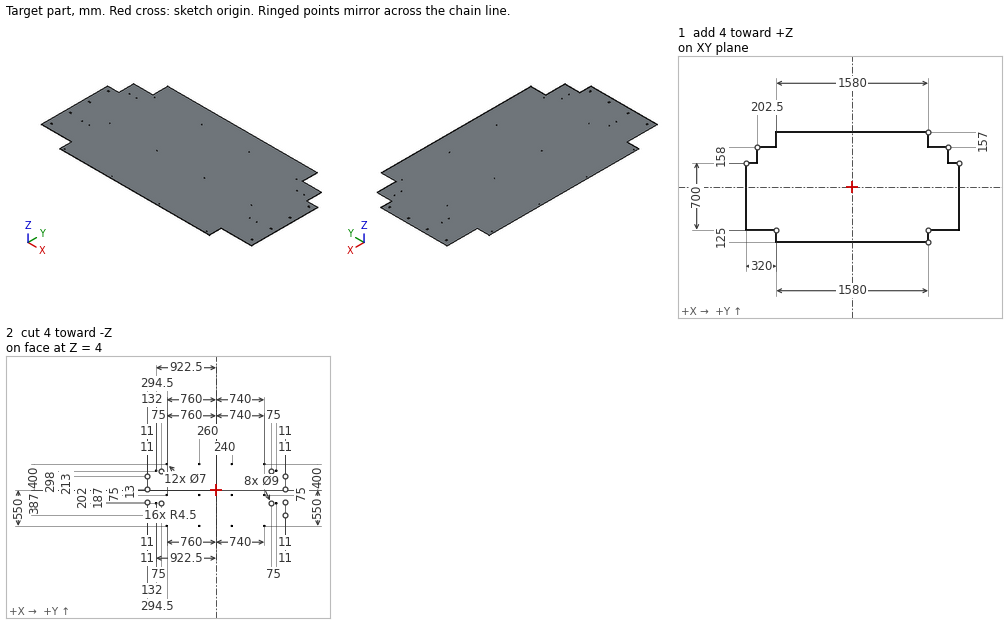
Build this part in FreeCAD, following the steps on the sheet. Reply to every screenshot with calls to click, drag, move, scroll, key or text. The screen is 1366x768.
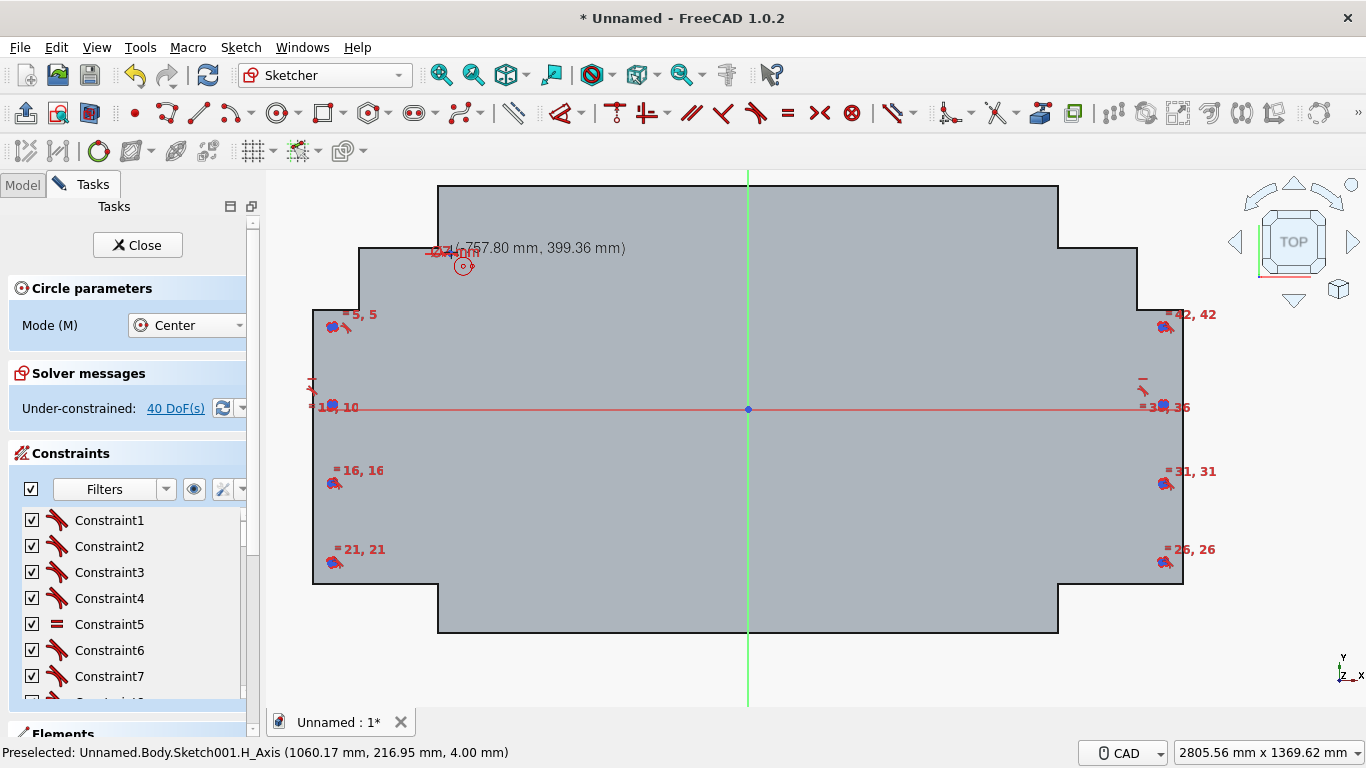
scroll(646, 253, up, 15)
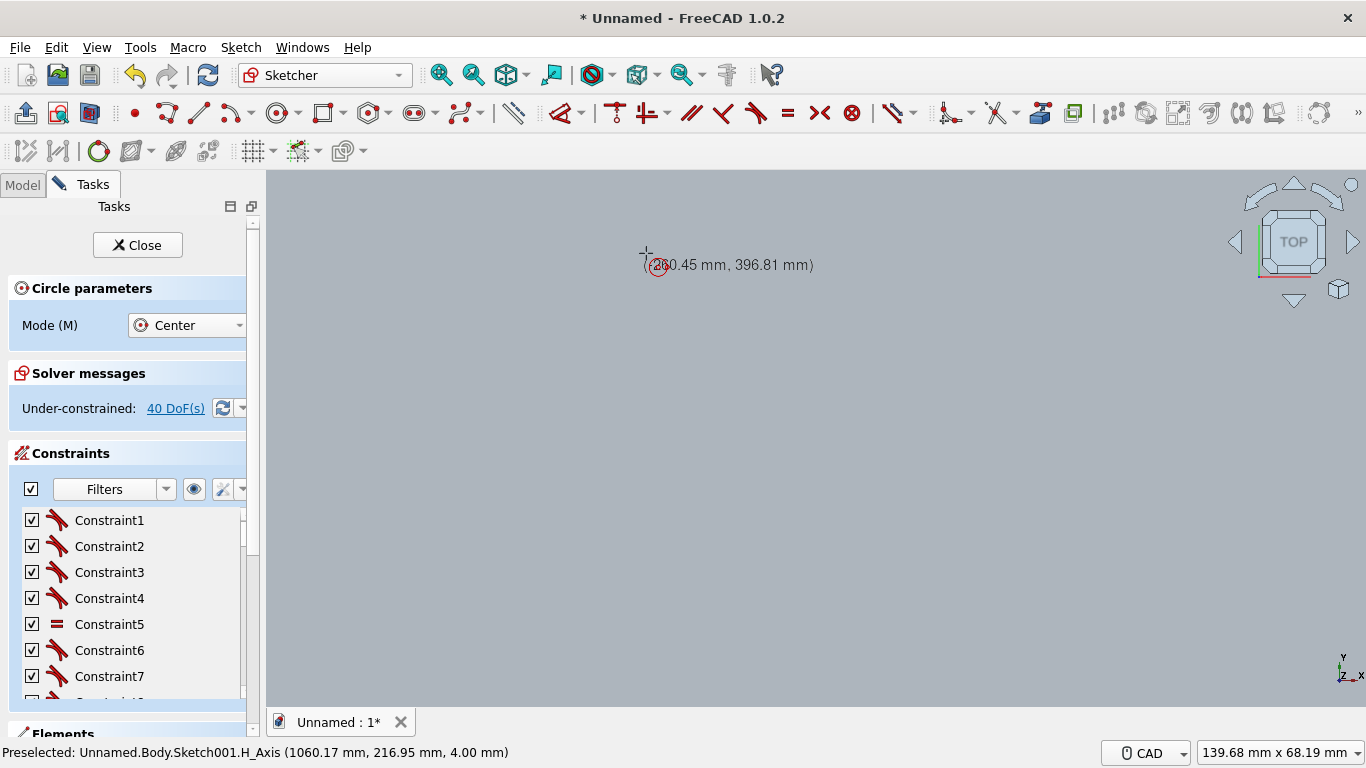
scroll(646, 253, down, 15)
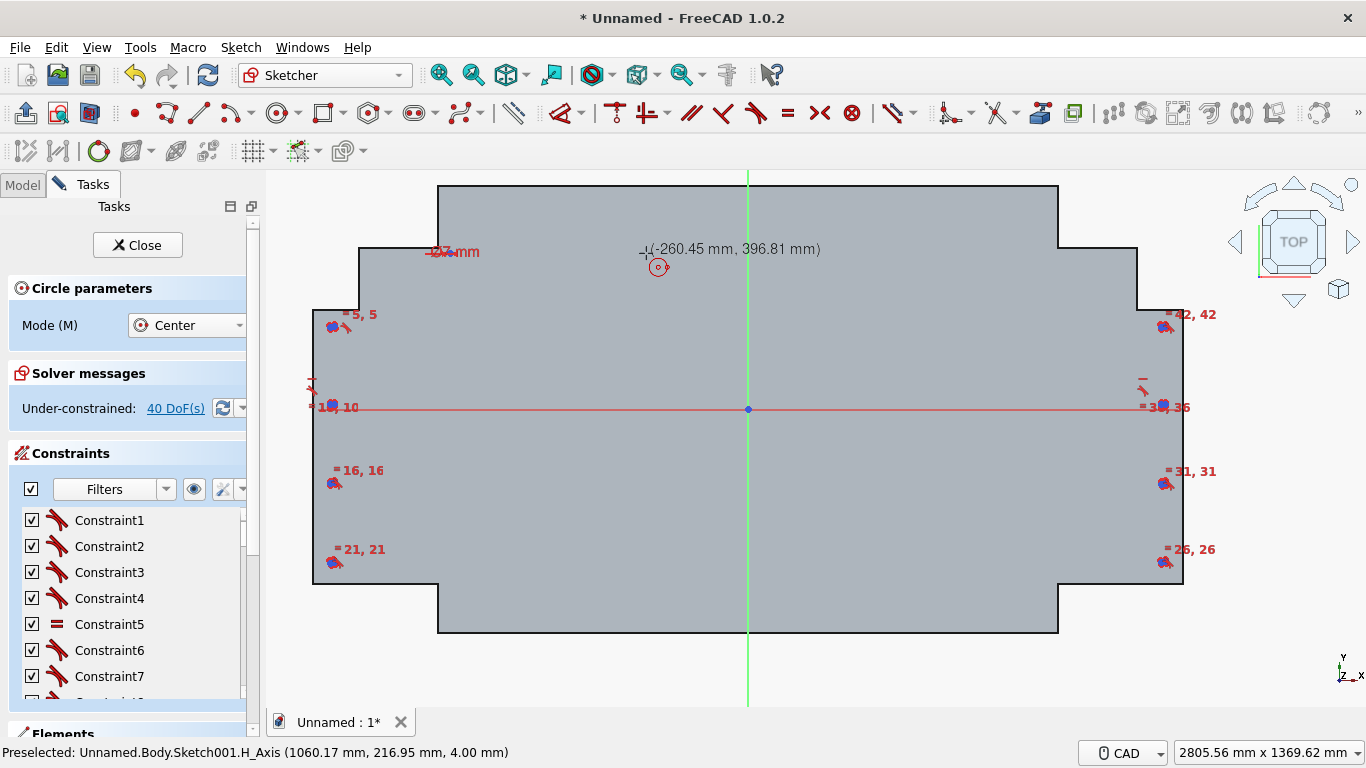
click(646, 253)
move(647, 252)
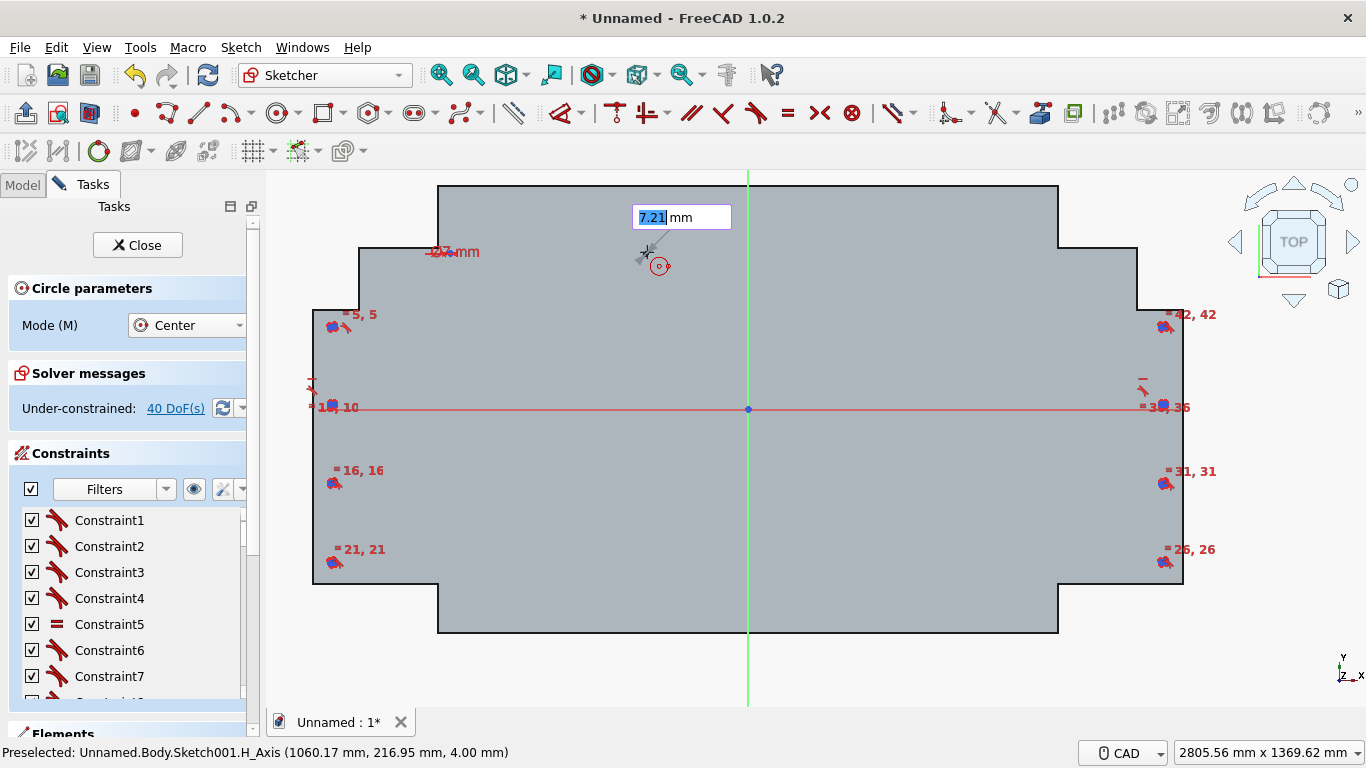
text(7)
key(Return)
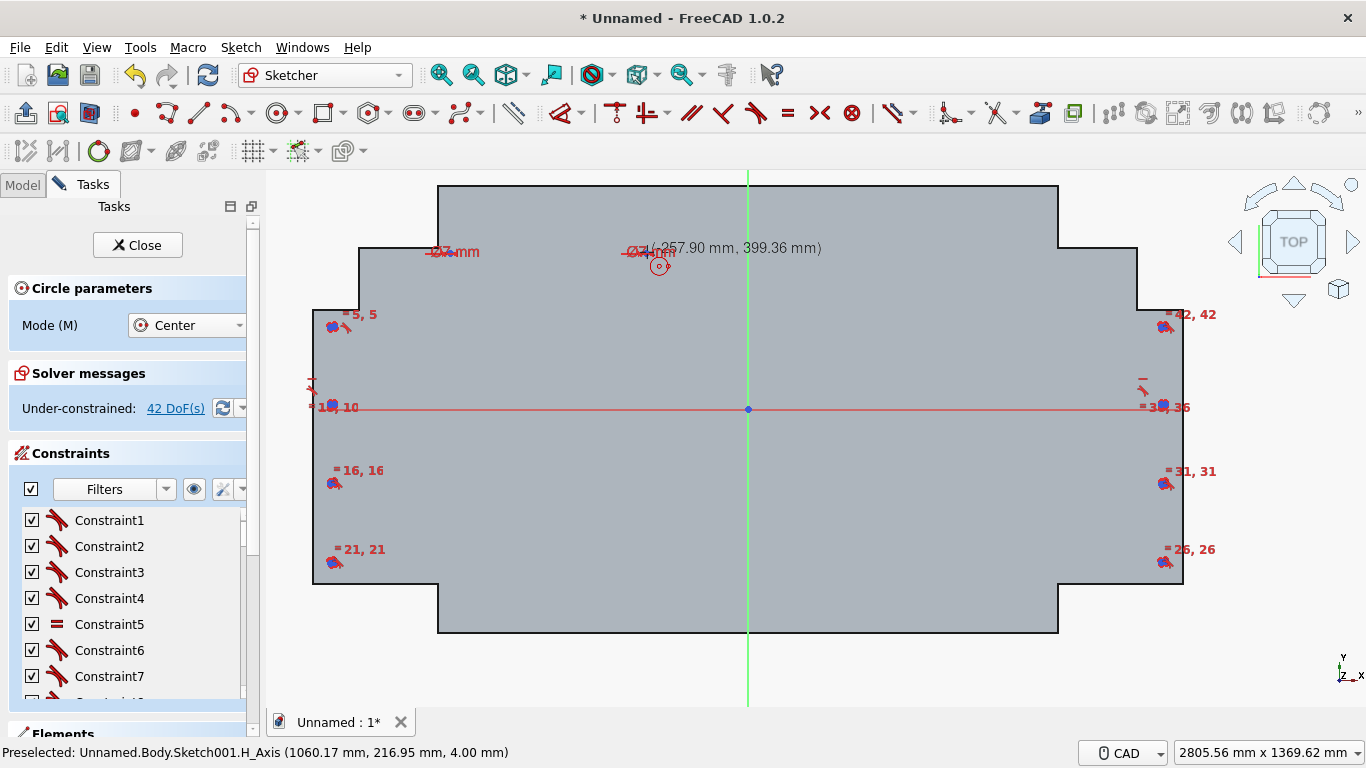
scroll(842, 253, up, 15)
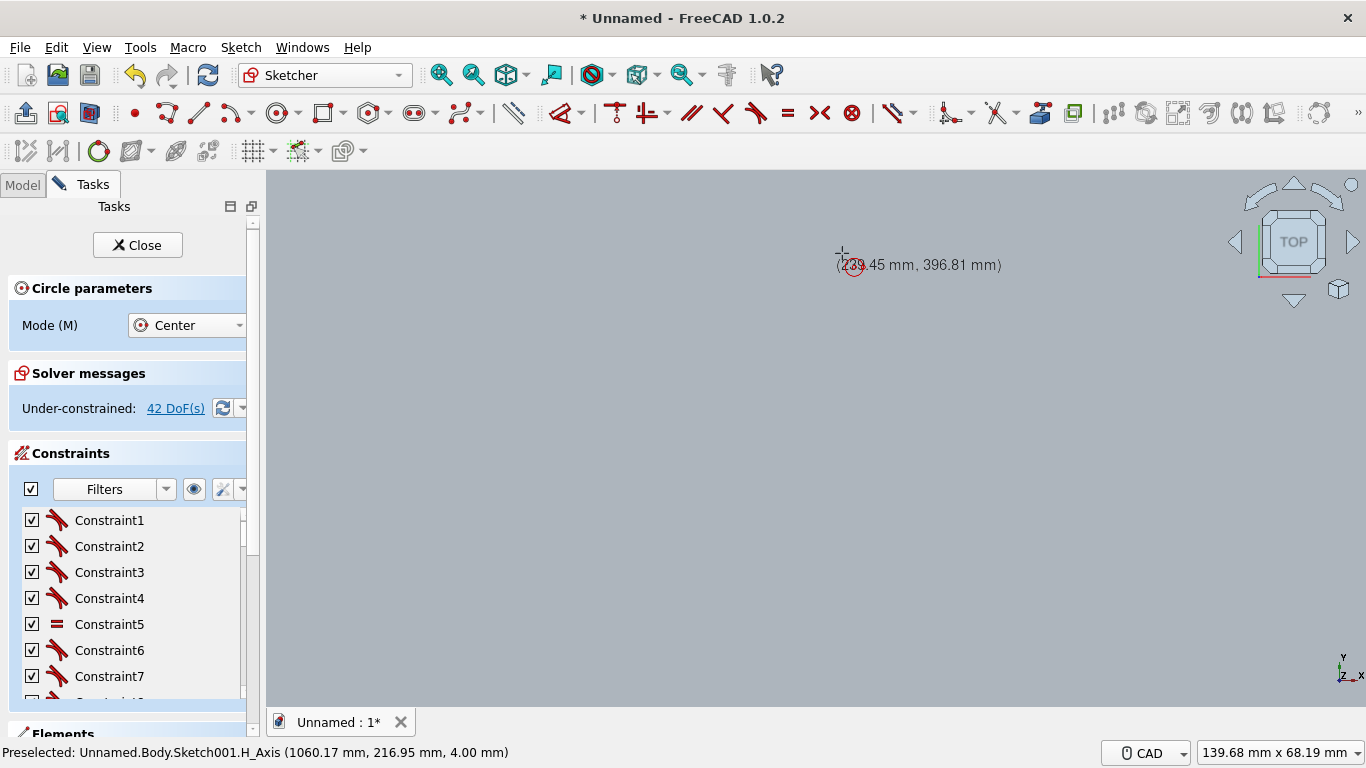
scroll(842, 253, down, 15)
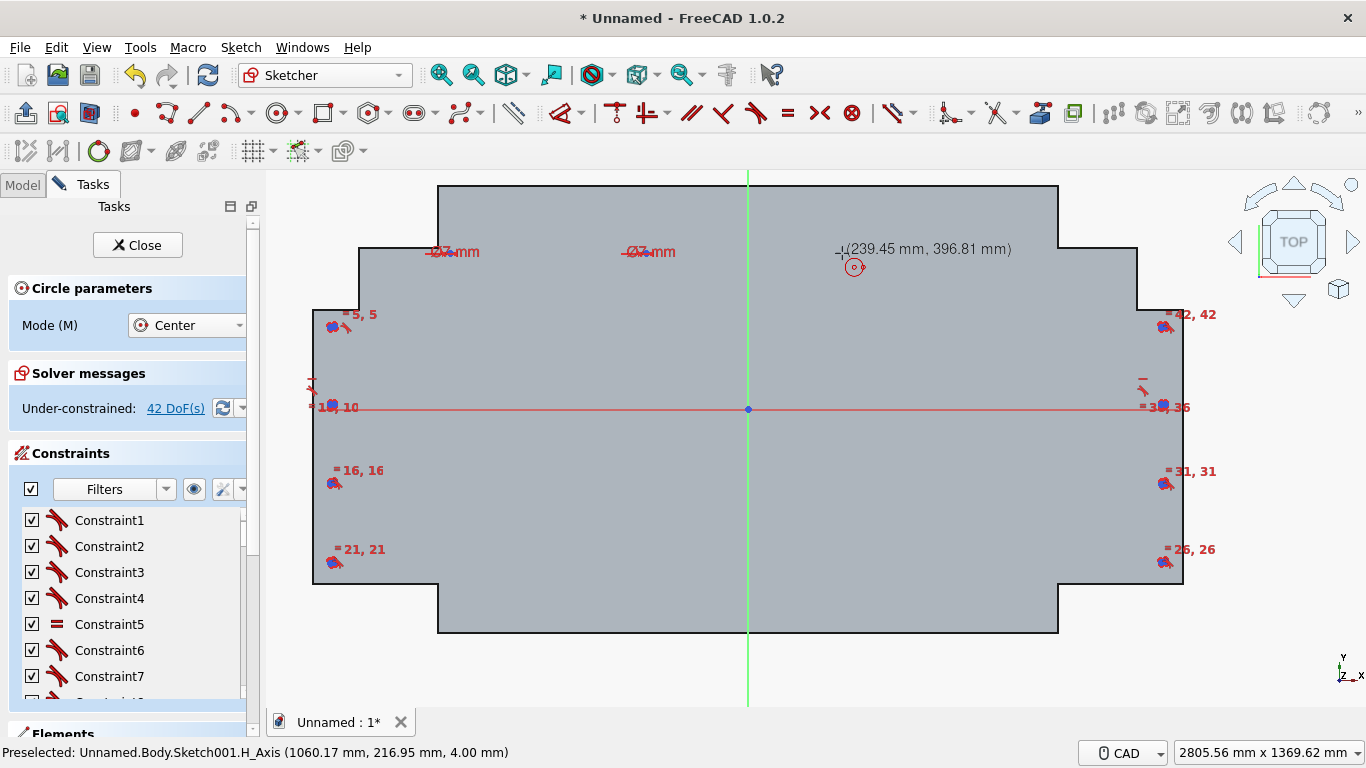
click(842, 253)
move(843, 252)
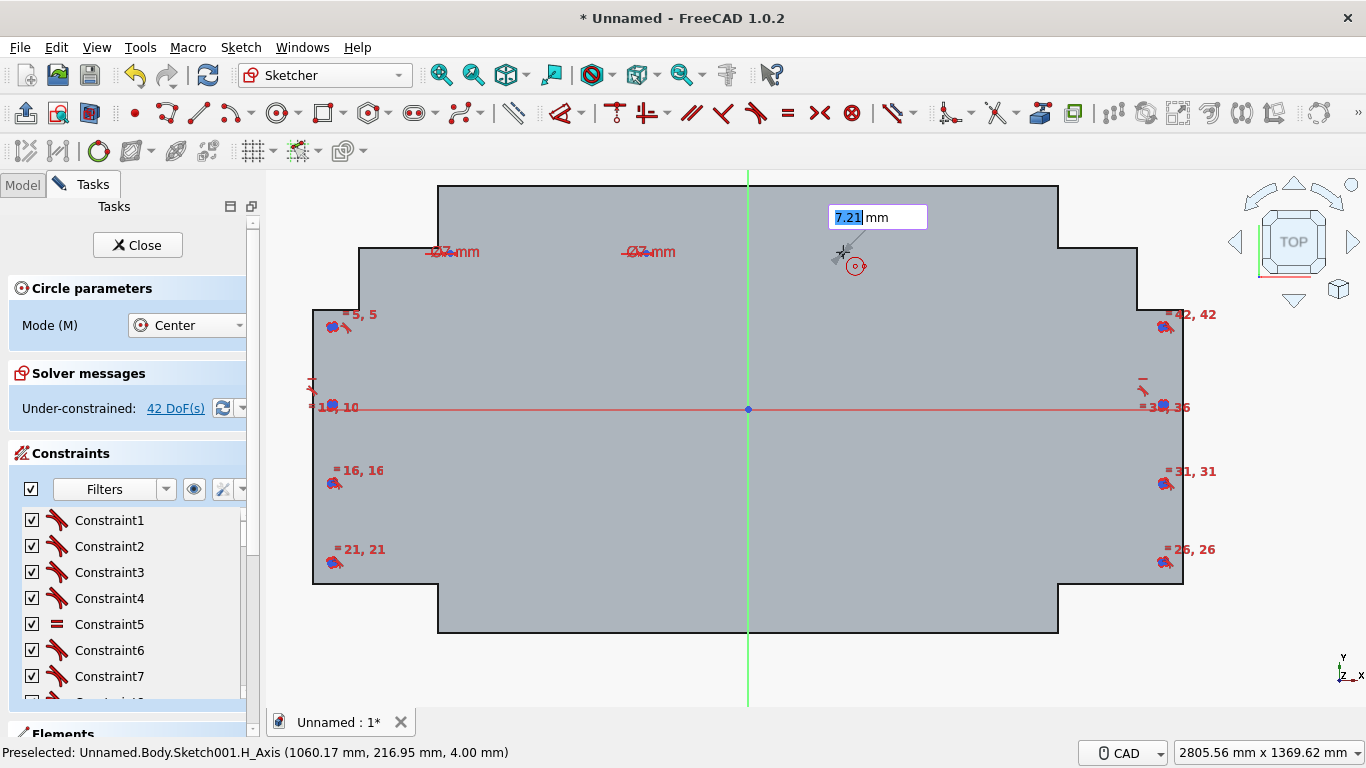
text(7)
key(Return)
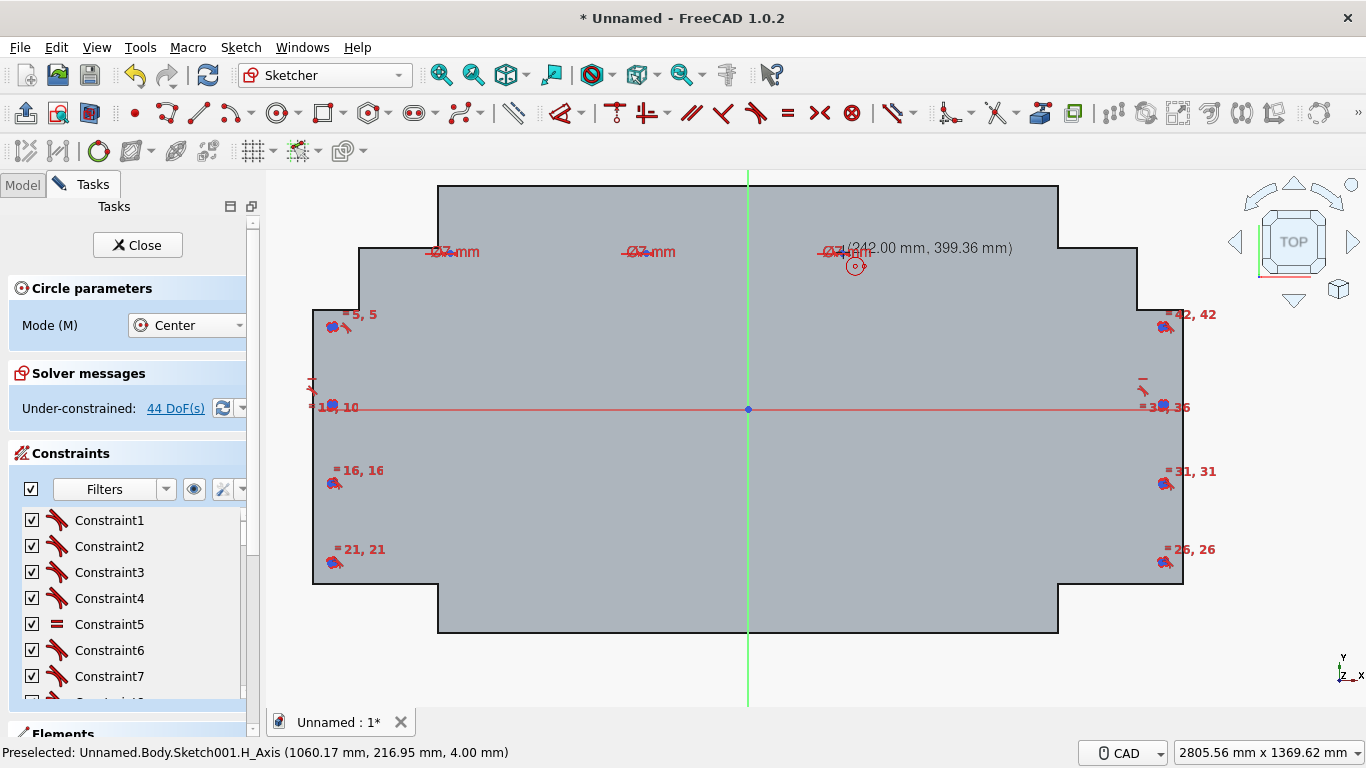
scroll(1038, 253, up, 15)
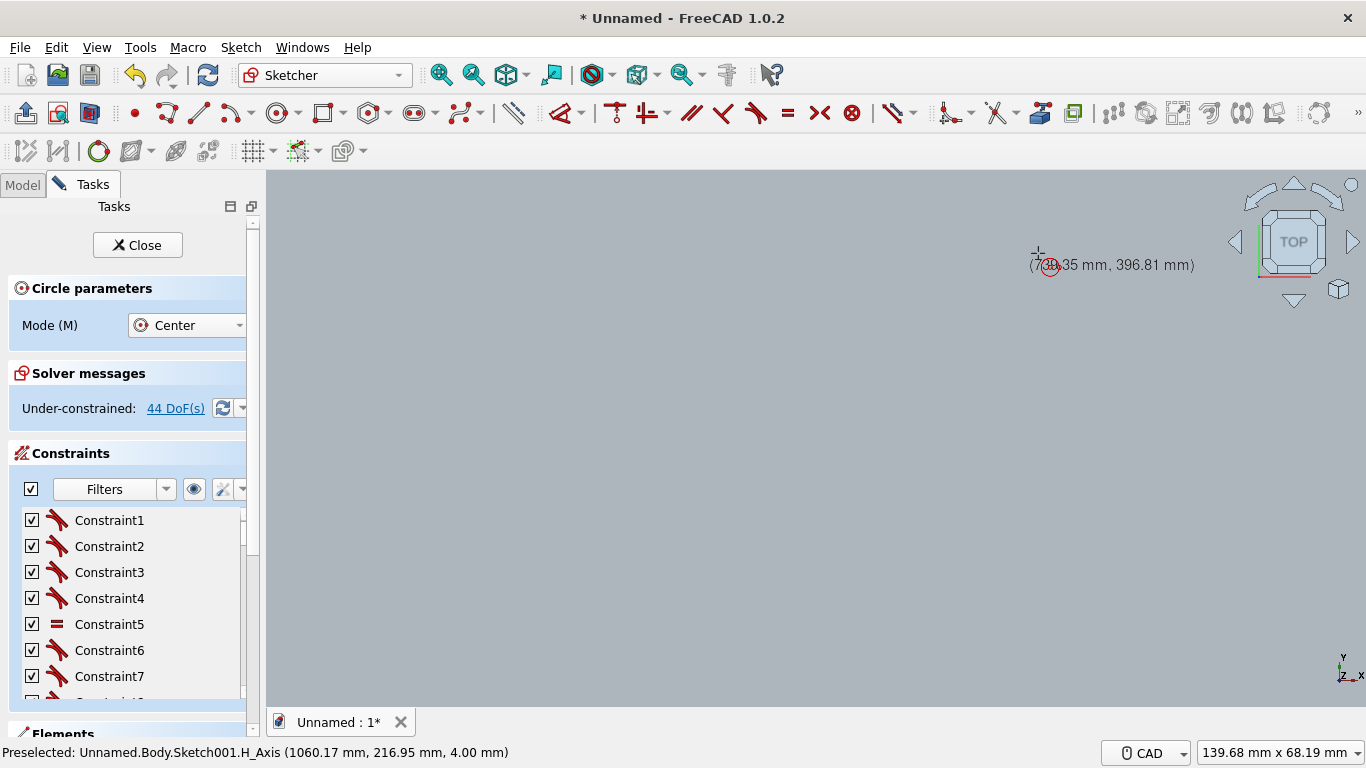
scroll(1038, 253, down, 15)